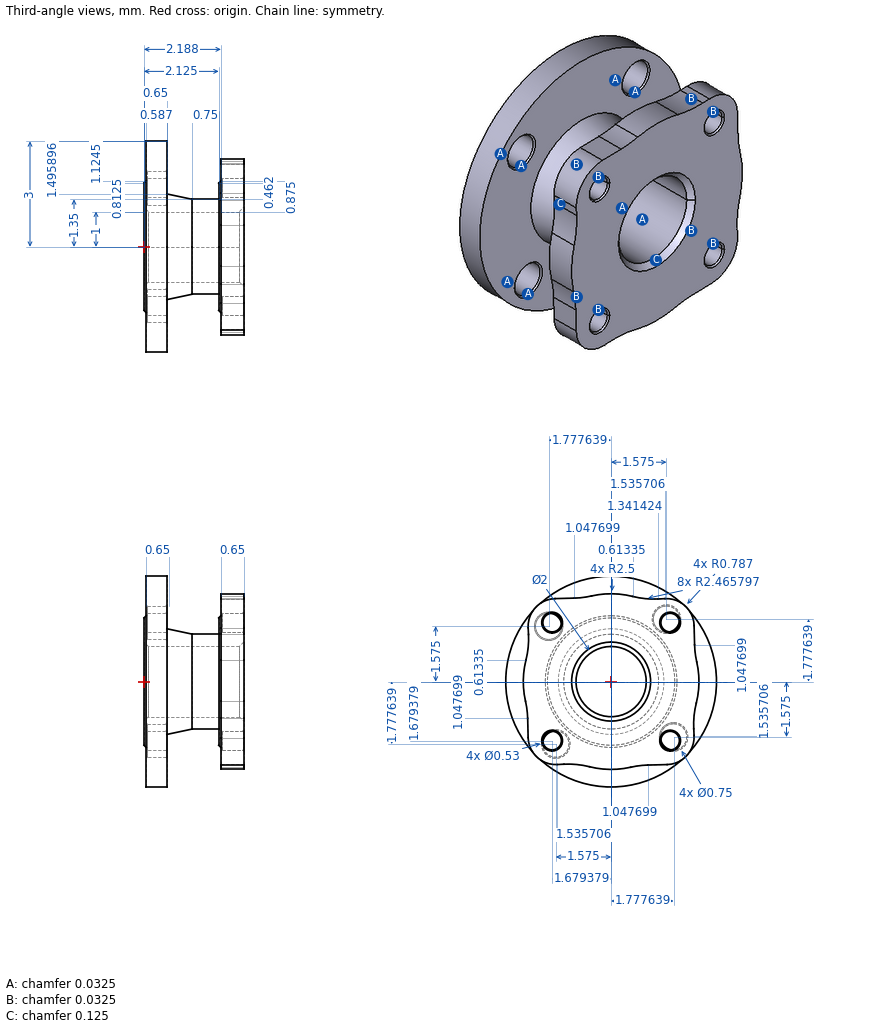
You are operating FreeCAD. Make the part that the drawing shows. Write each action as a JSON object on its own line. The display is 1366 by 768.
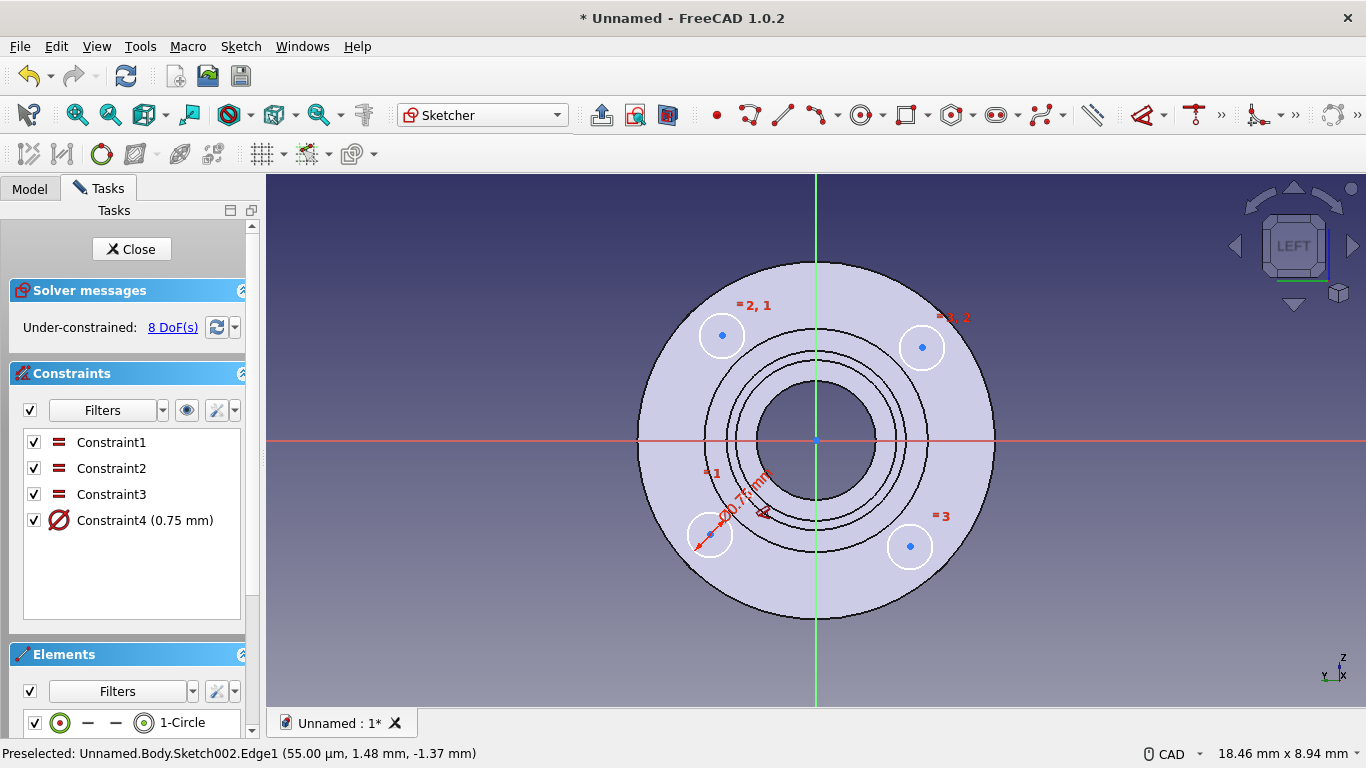
{"action": "left_click", "coordinate": [710, 535]}
{"action": "left_click", "coordinate": [676, 488]}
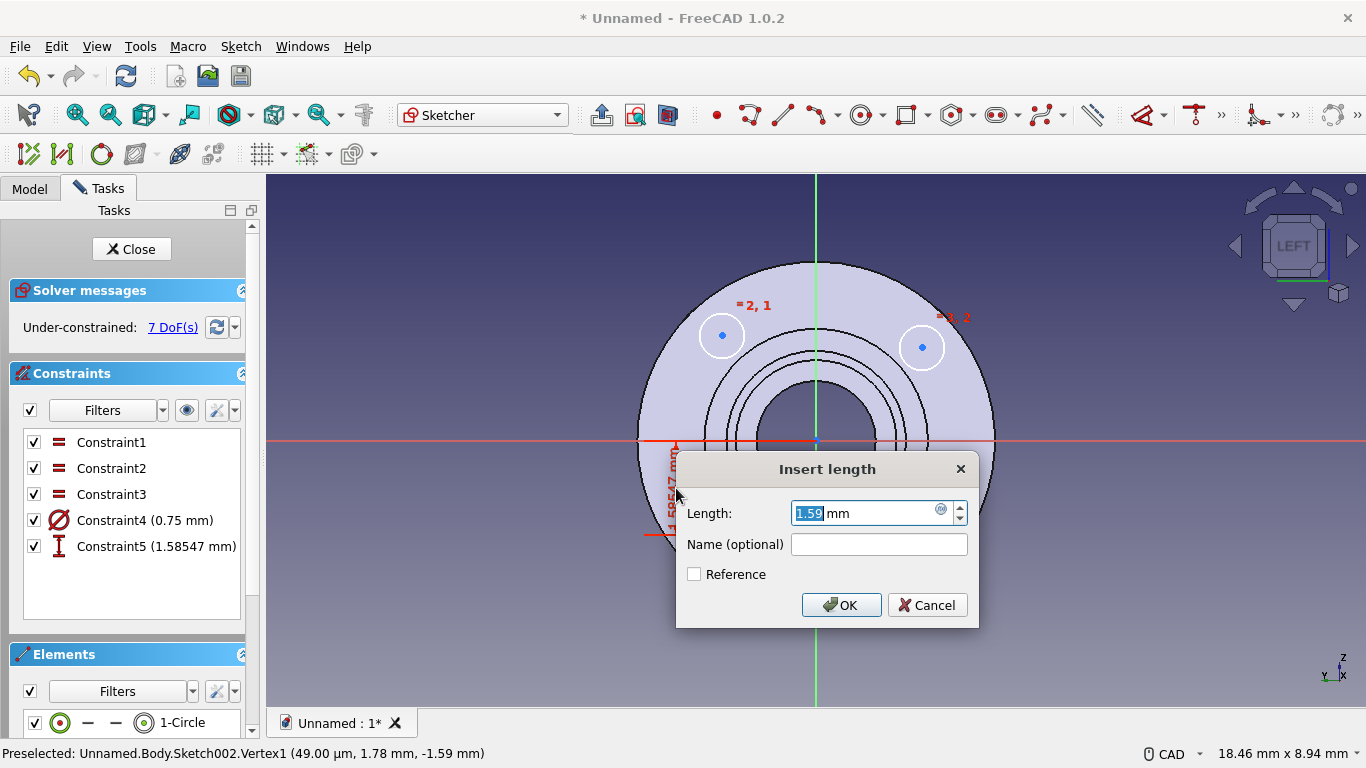
{"action": "type", "text": "1.575"}
{"action": "key", "text": "Return"}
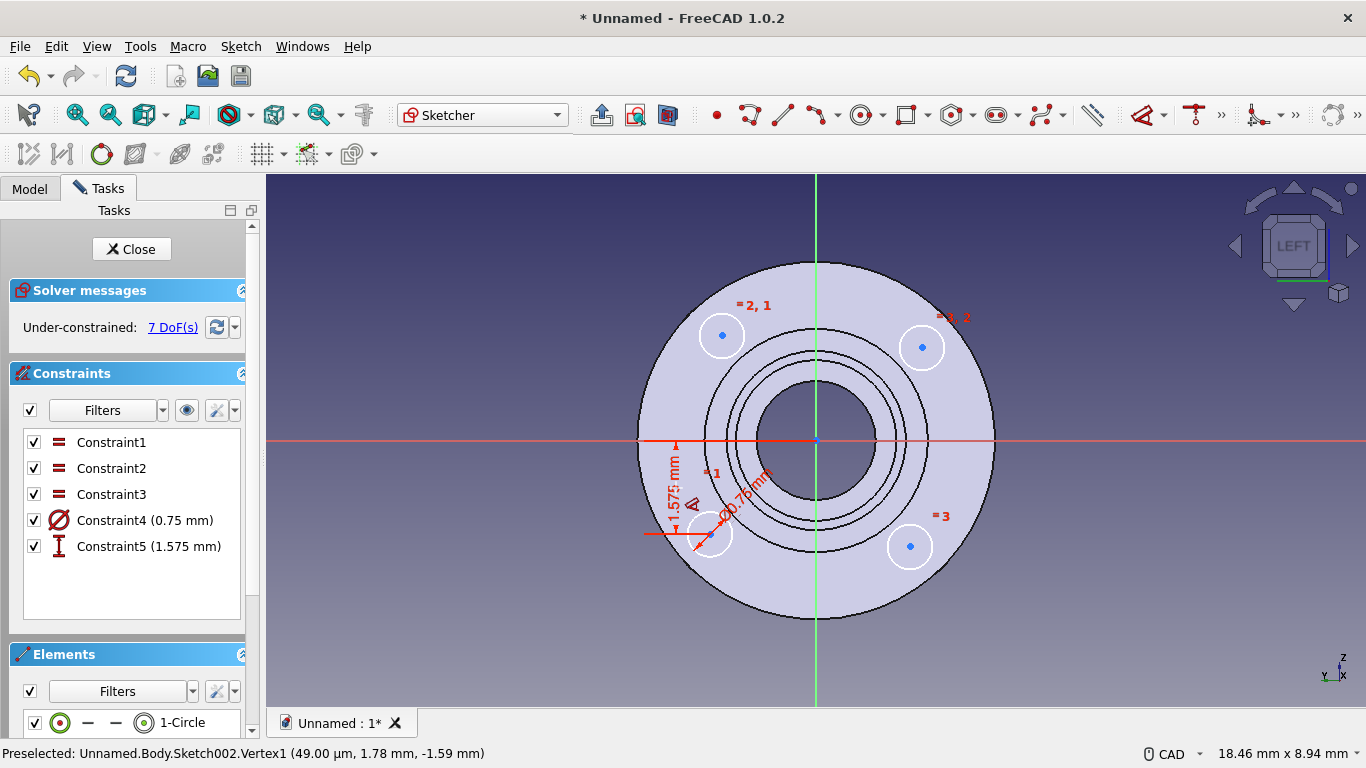
{"action": "left_click", "coordinate": [722, 336]}
{"action": "left_click", "coordinate": [769, 302]}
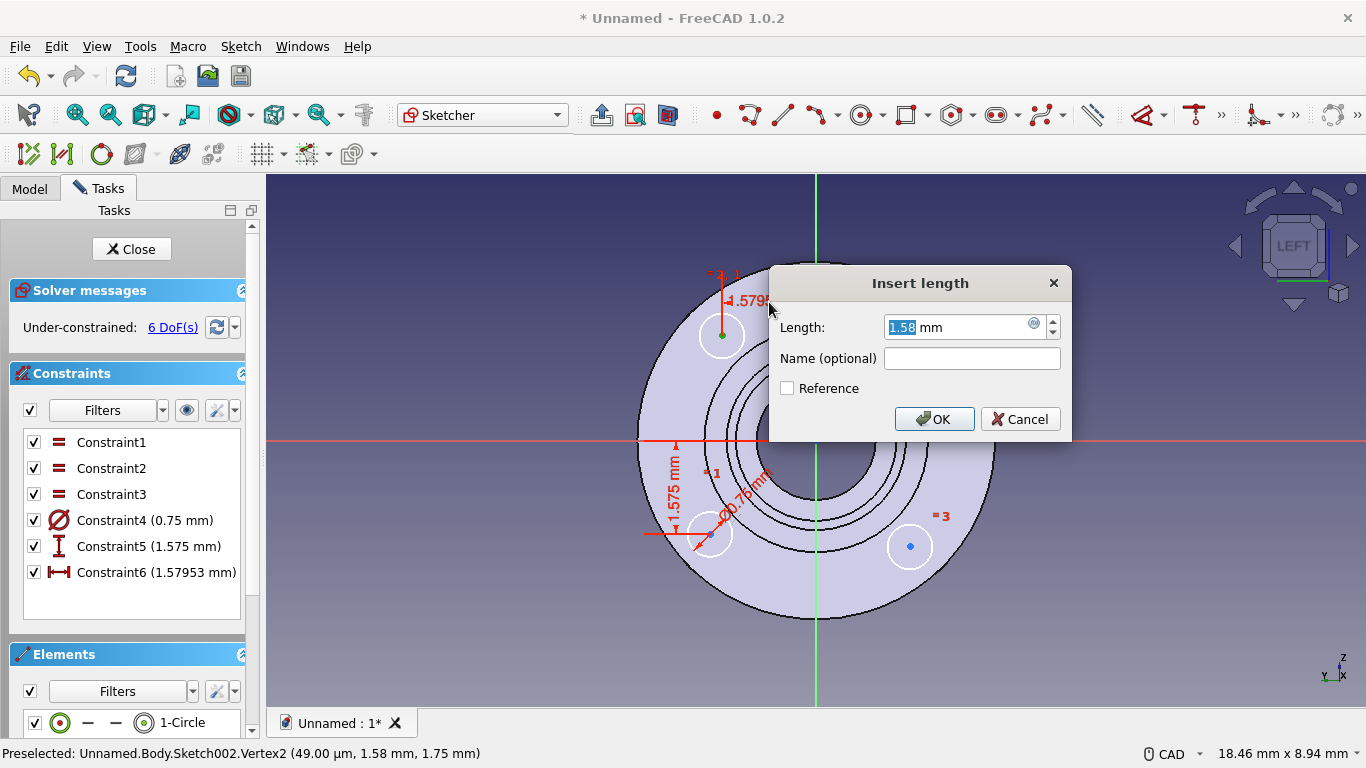
{"action": "type", "text": "1.575"}
{"action": "key", "text": "Return"}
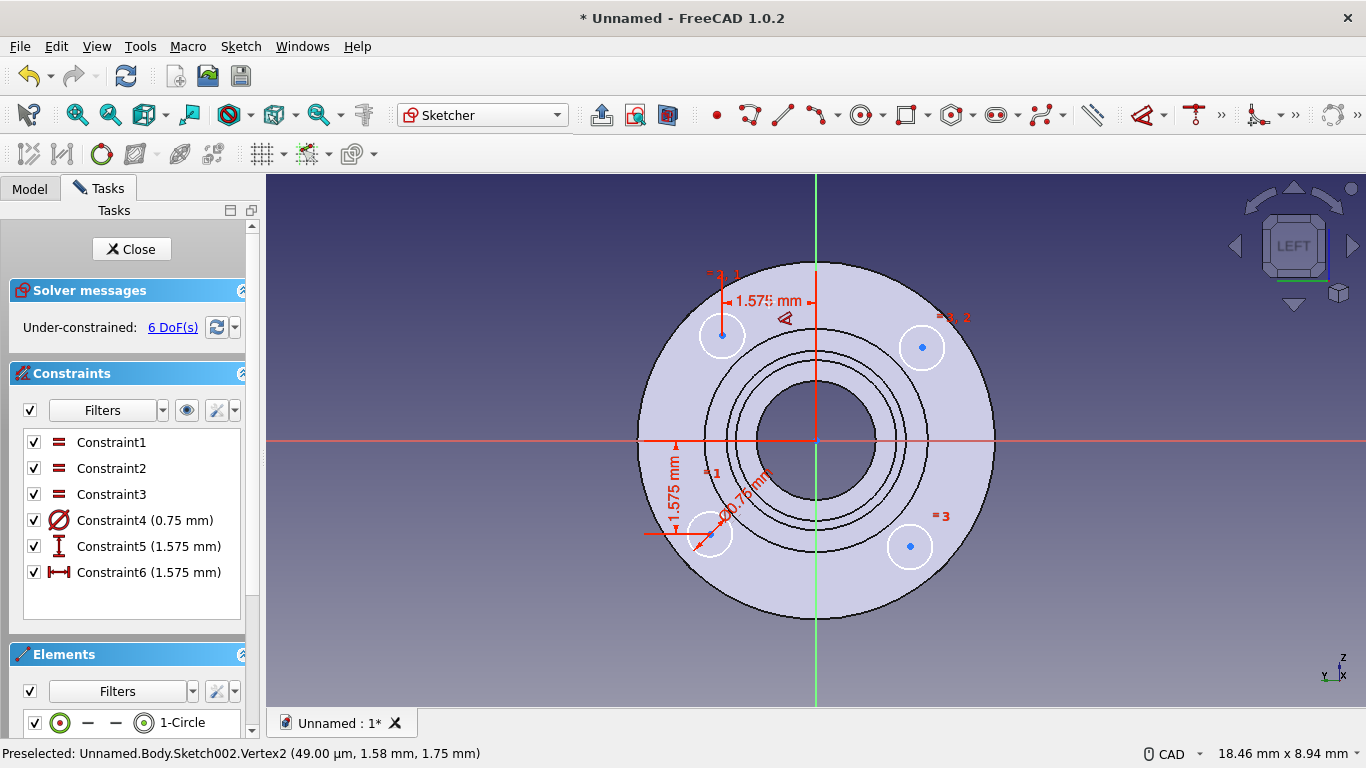
{"action": "left_click", "coordinate": [922, 348]}
{"action": "left_click", "coordinate": [956, 394]}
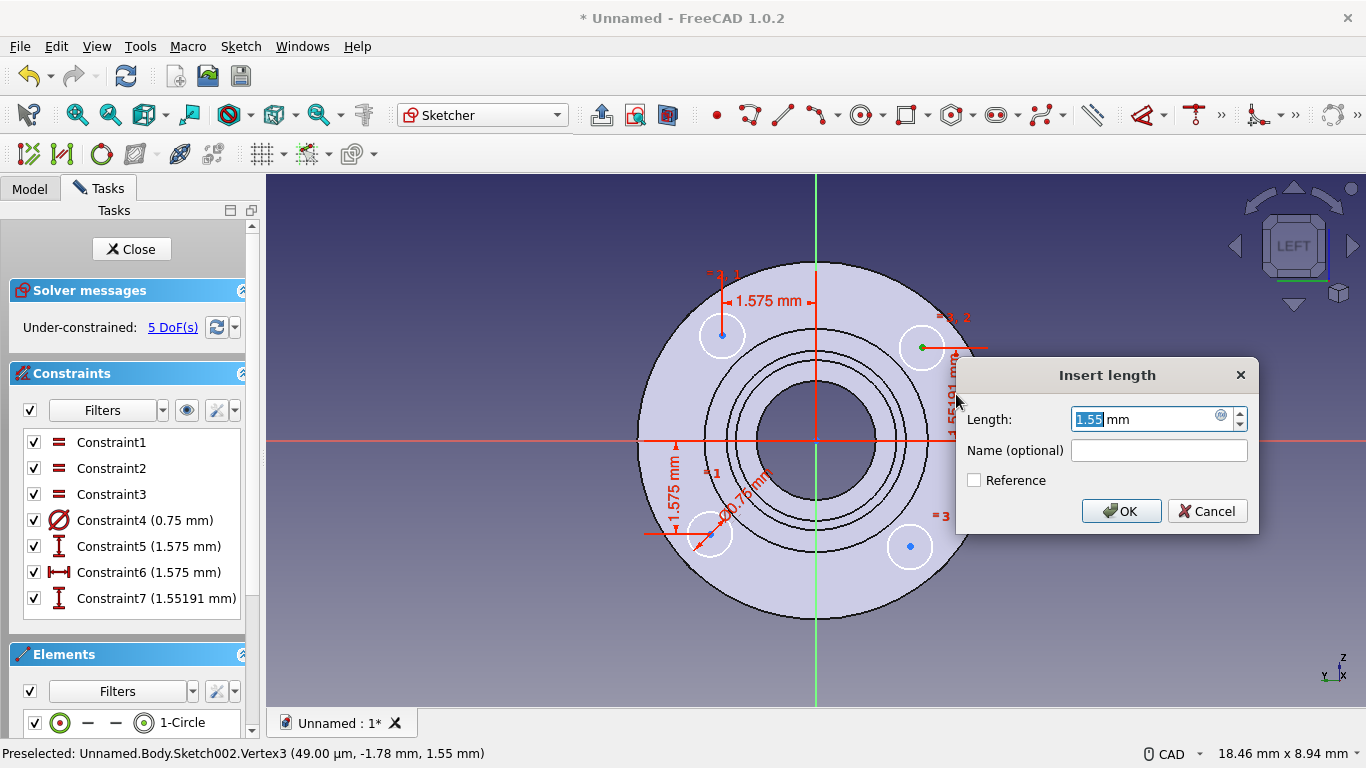
{"action": "type", "text": "1.575"}
{"action": "key", "text": "Return"}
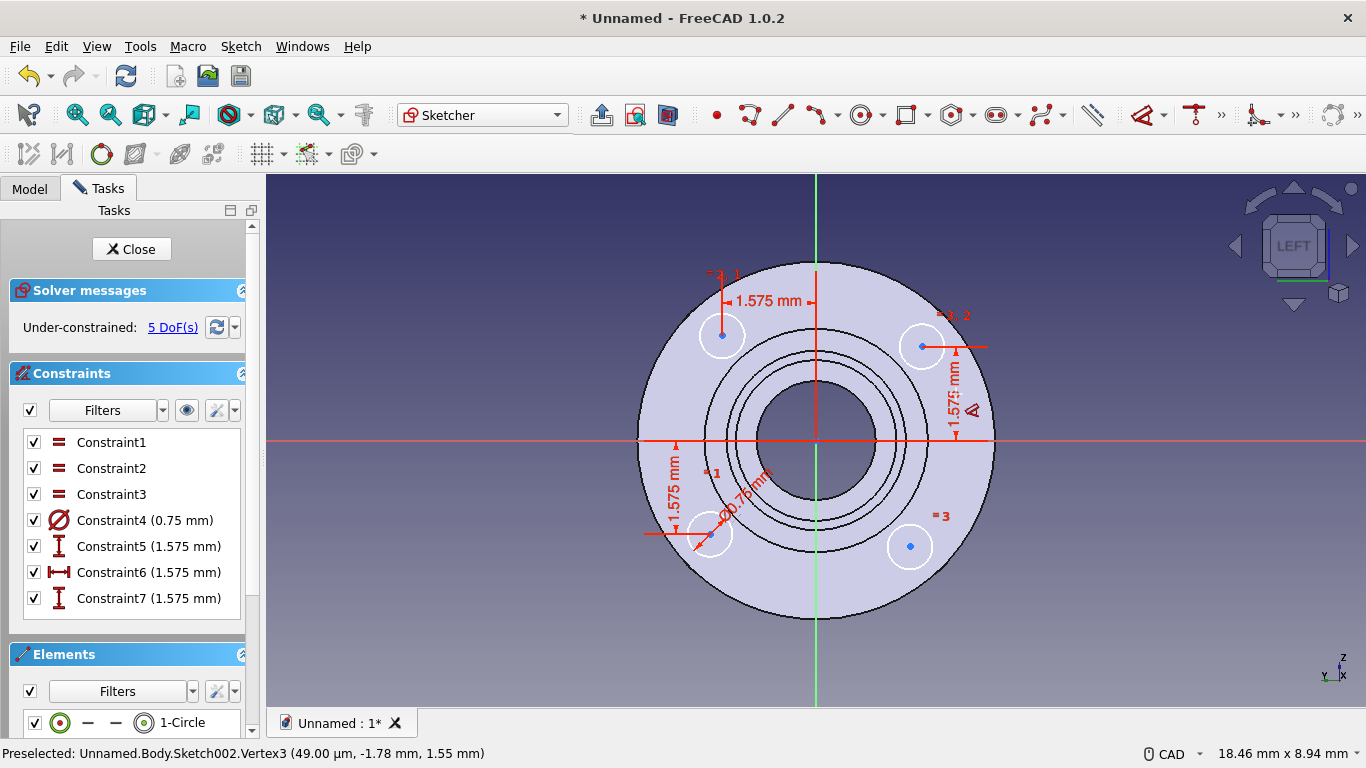
{"action": "left_click", "coordinate": [910, 547]}
{"action": "left_click", "coordinate": [863, 581]}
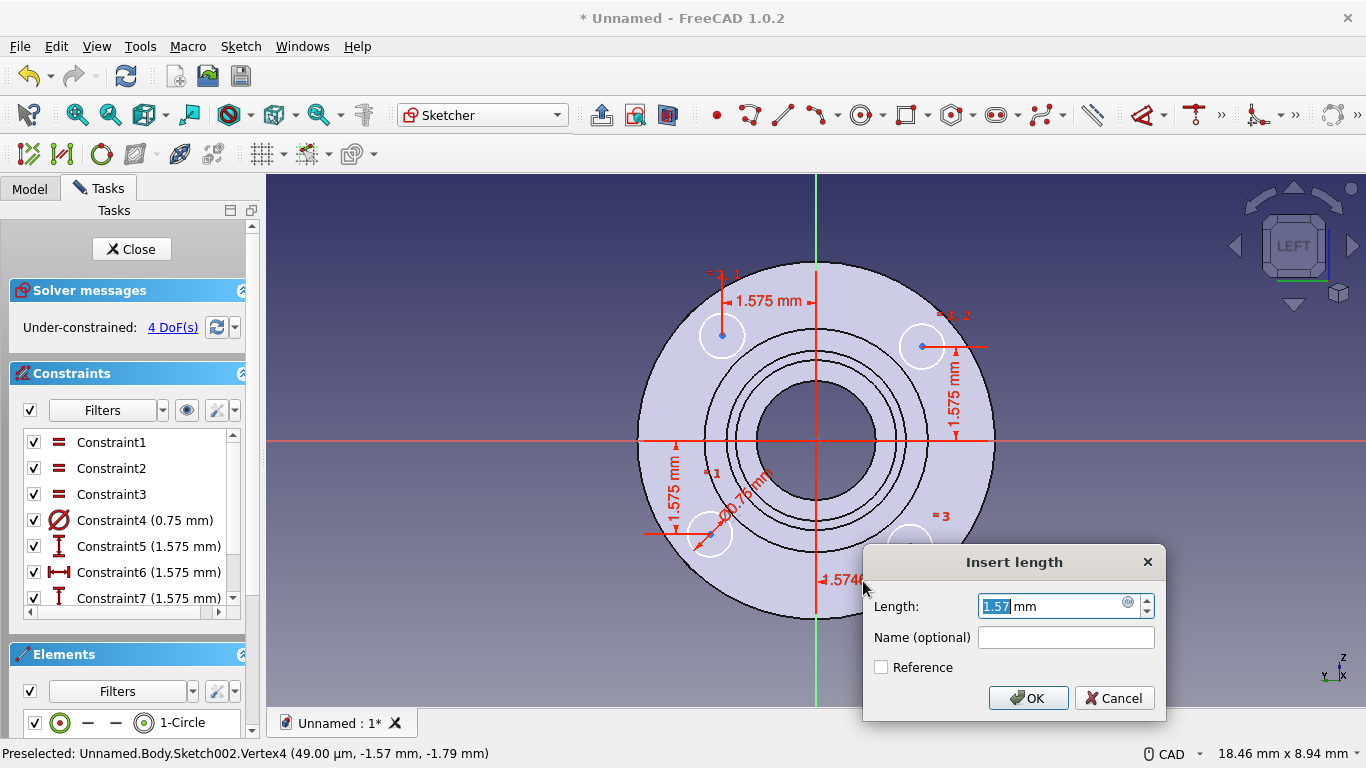
{"action": "type", "text": "1.575"}
{"action": "key", "text": "Return"}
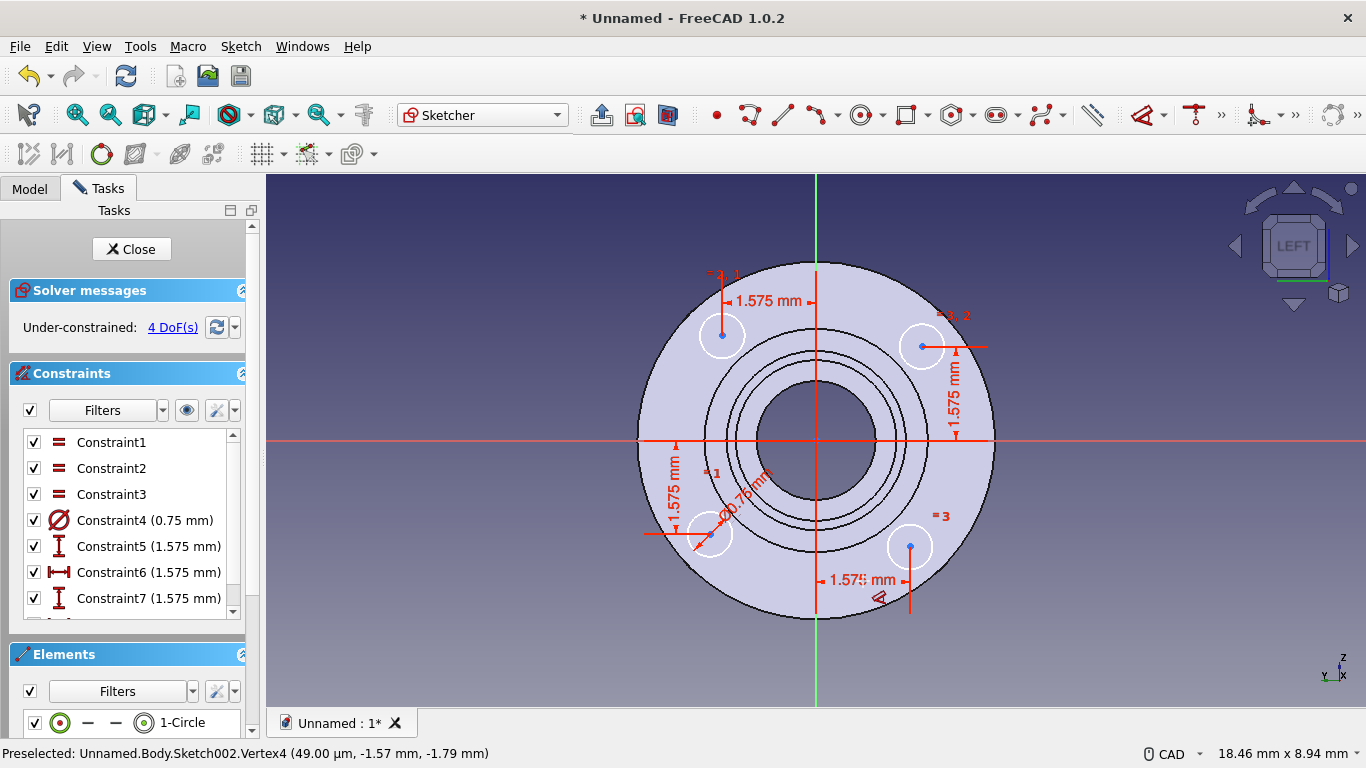
{"action": "left_click", "coordinate": [710, 534]}
{"action": "left_click", "coordinate": [763, 568]}